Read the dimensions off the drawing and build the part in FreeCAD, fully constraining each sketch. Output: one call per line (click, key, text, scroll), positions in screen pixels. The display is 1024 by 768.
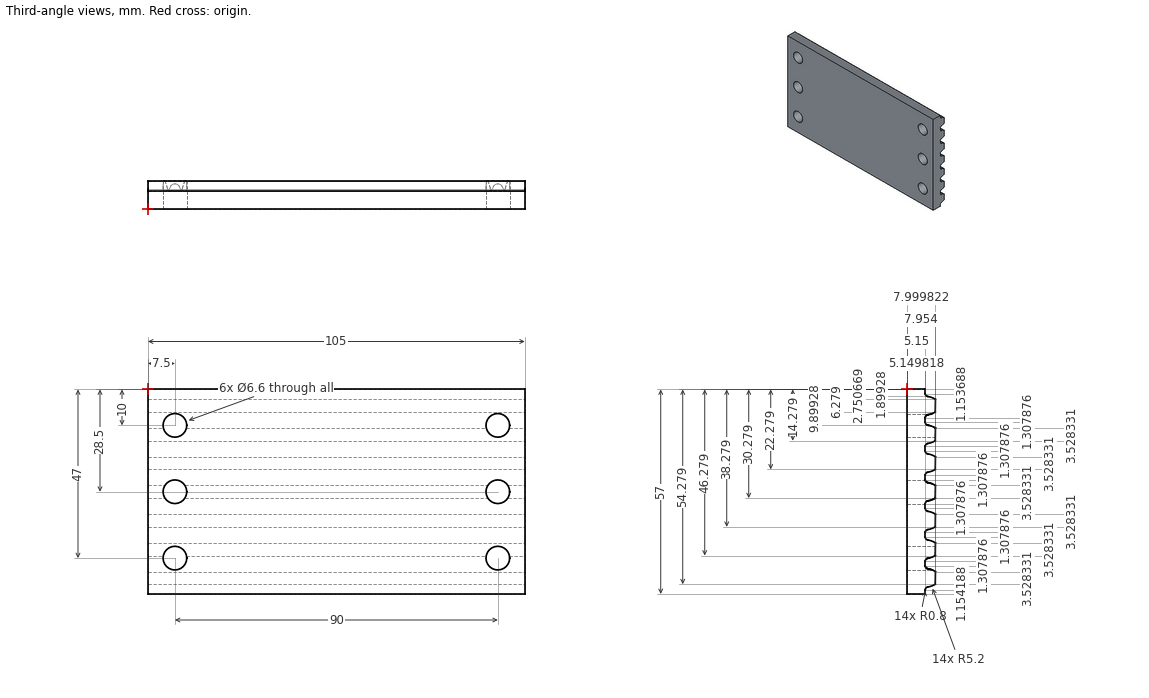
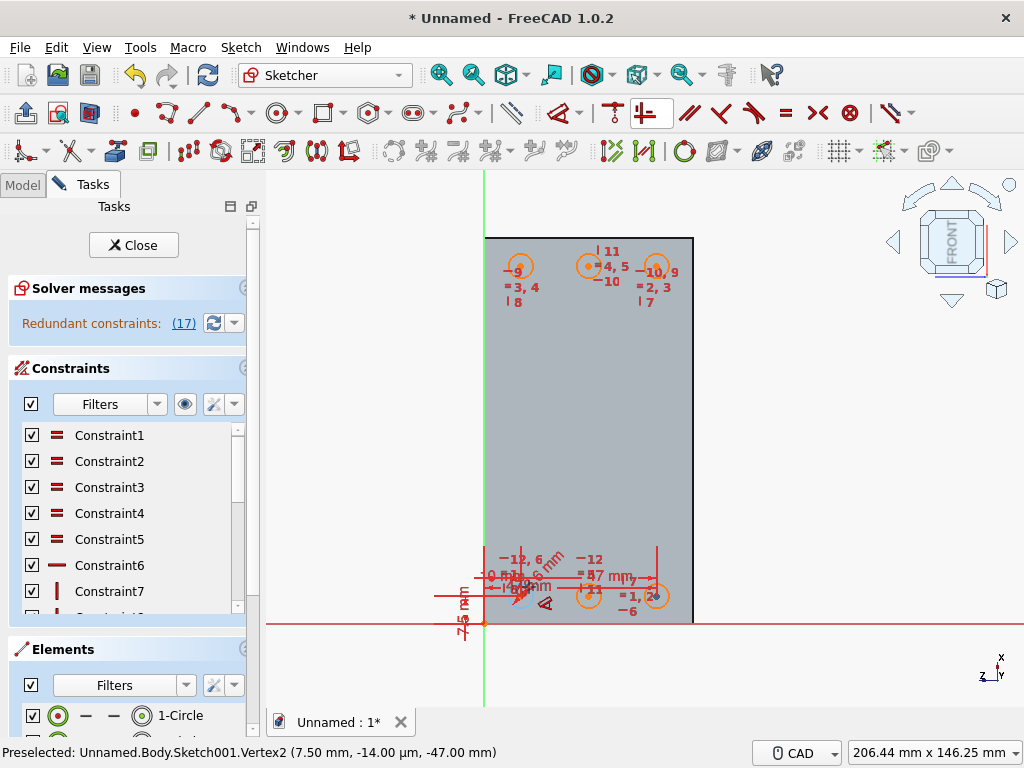
click(657, 266)
click(691, 431)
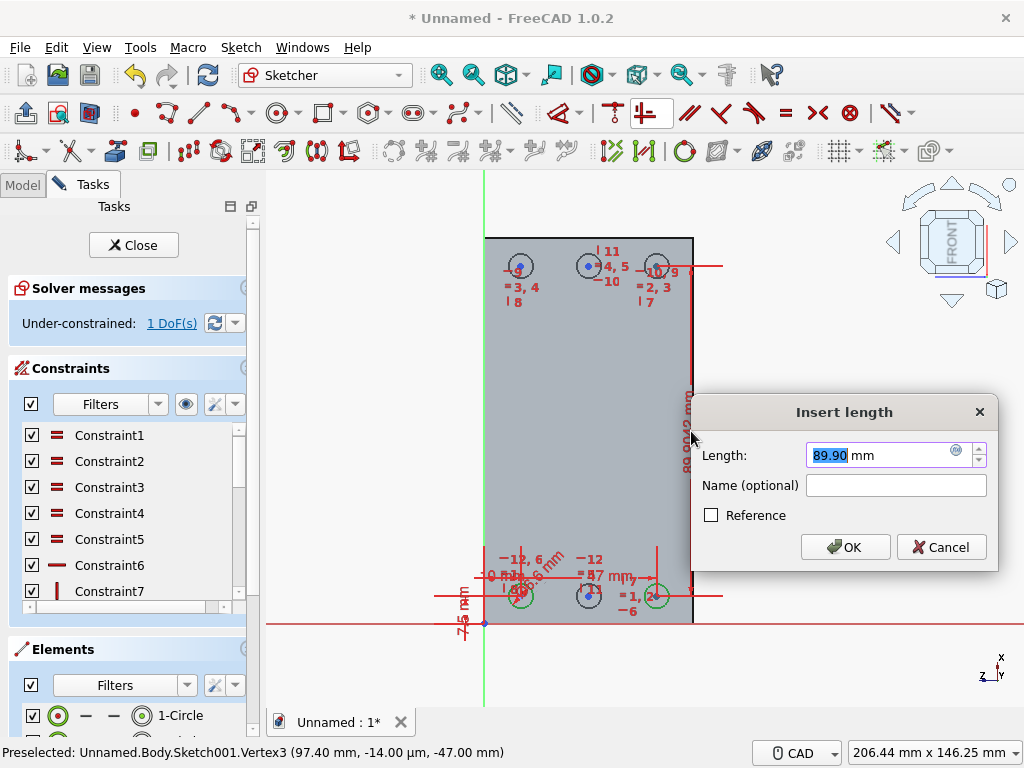
text(90)
key(Return)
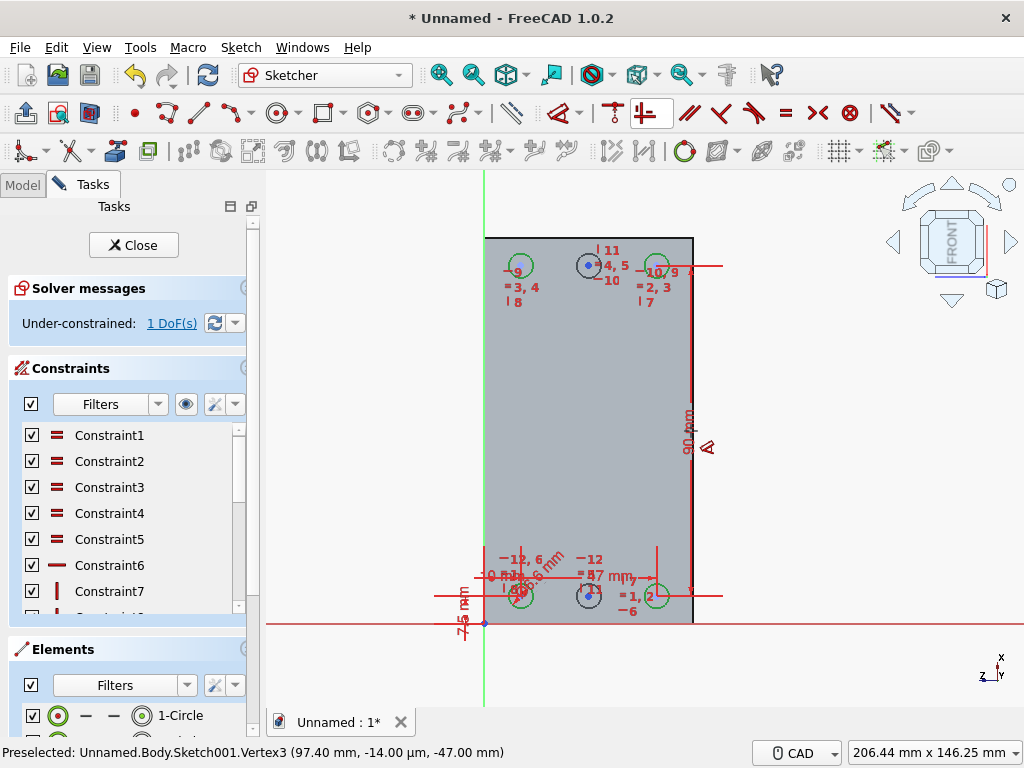
click(589, 266)
click(537, 658)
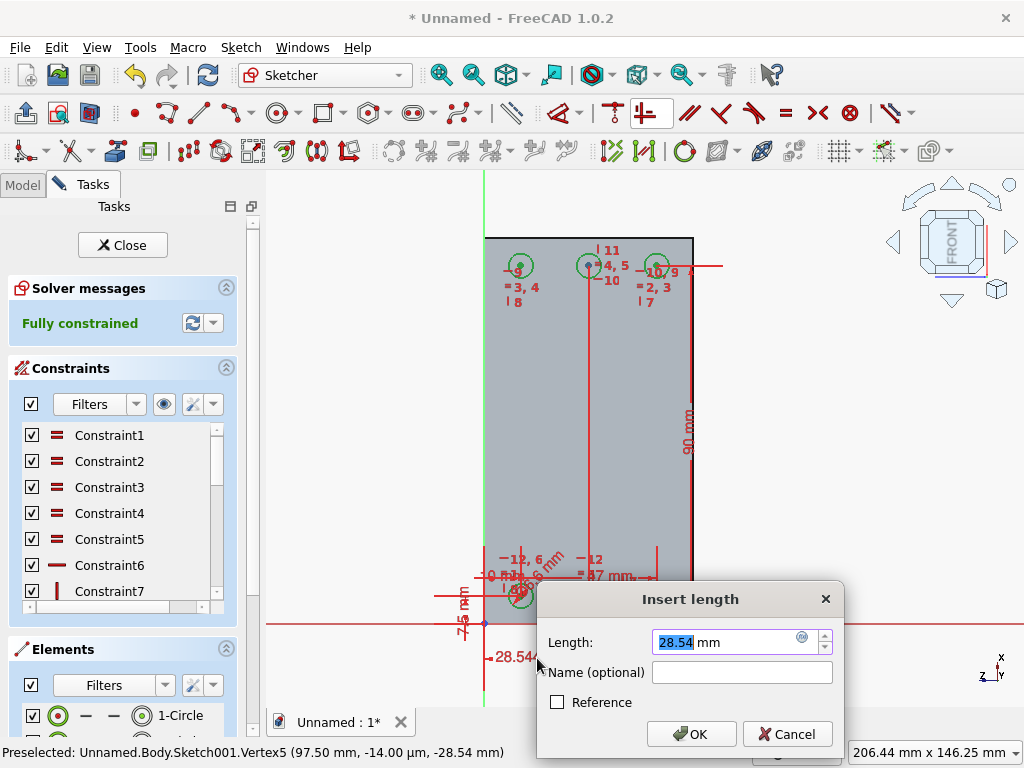
text(28.5)
key(Return)
key(Escape)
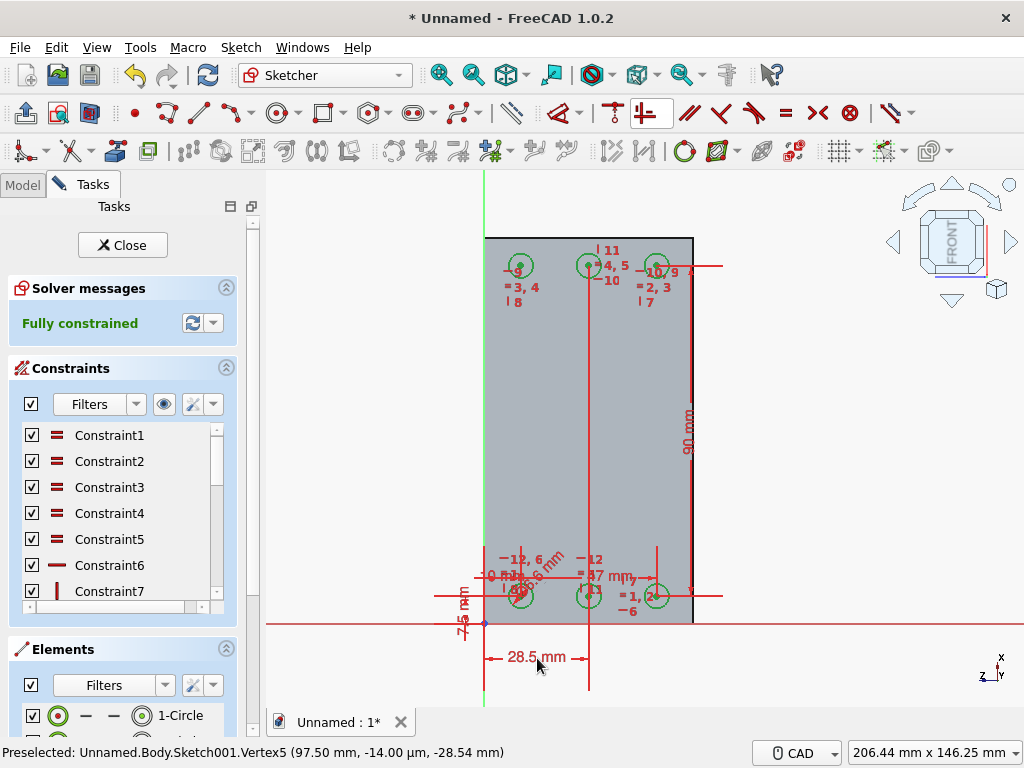
click(123, 245)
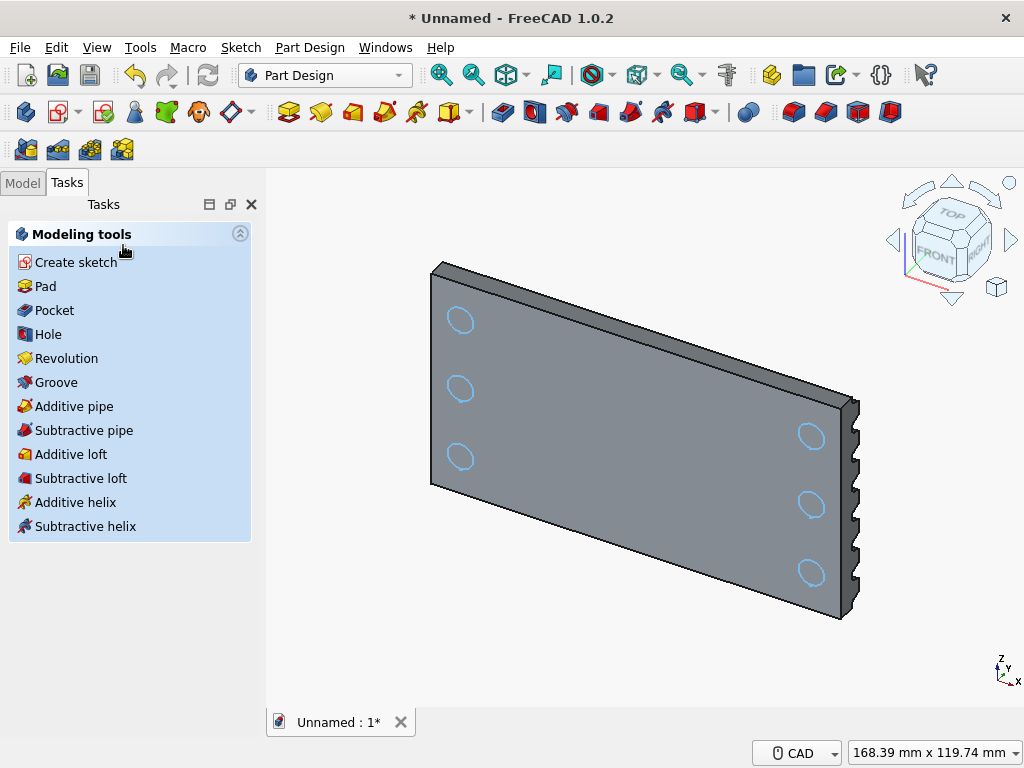
click(536, 112)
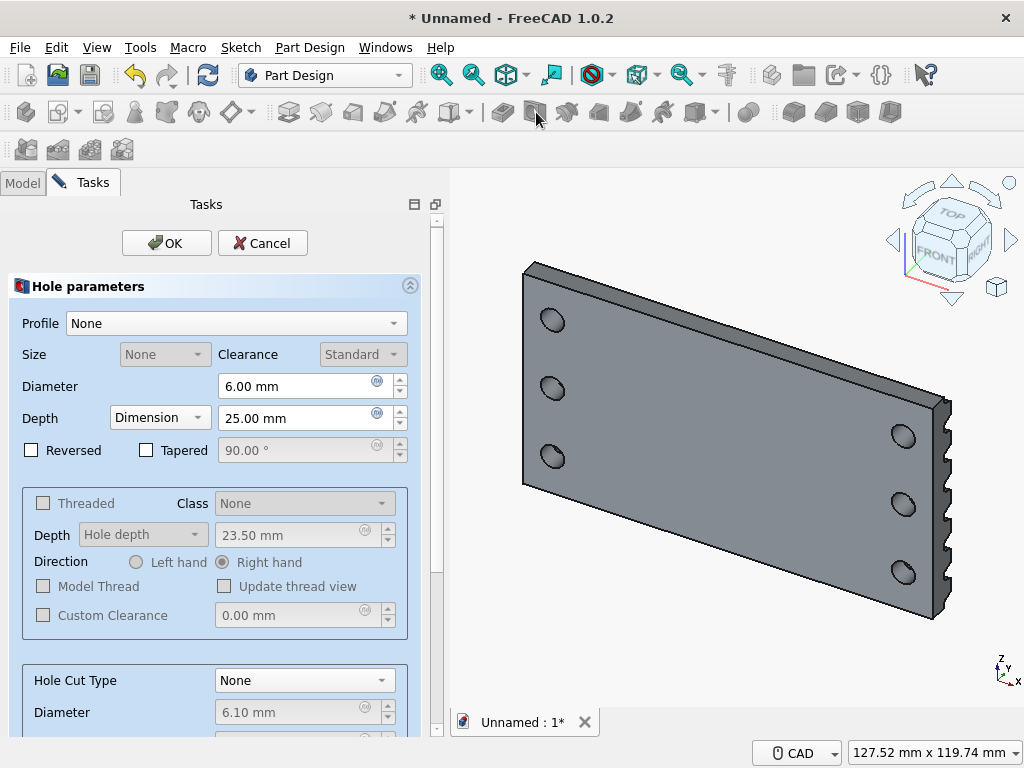
triple_click(305, 386)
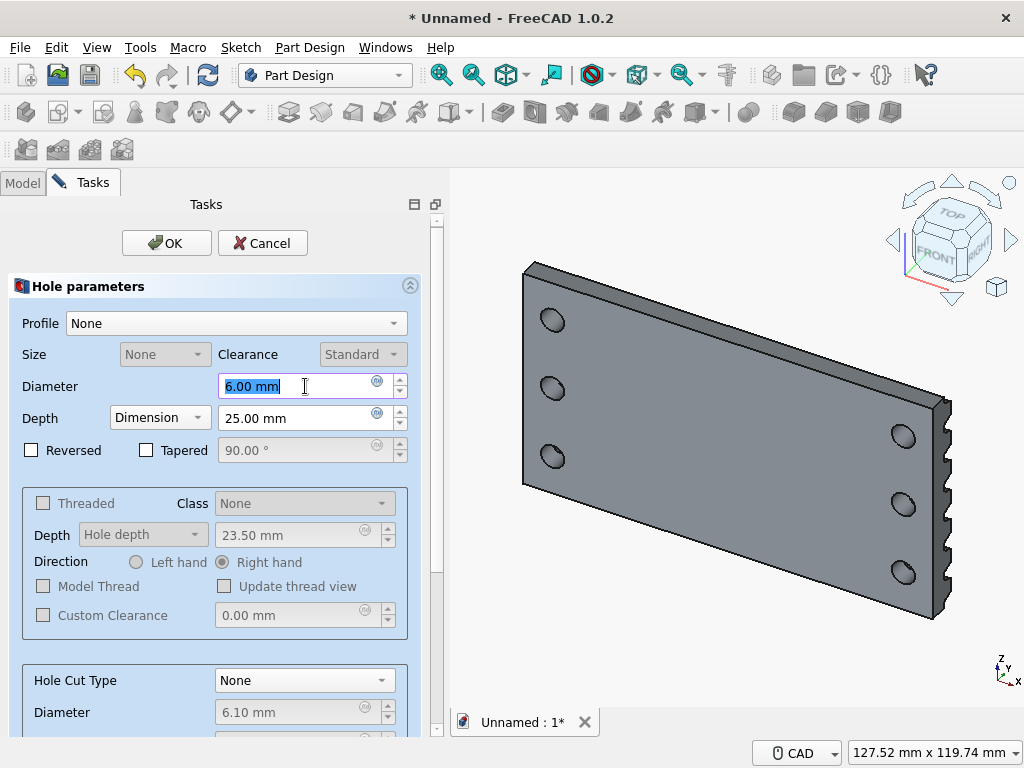
text(6.6)
key(Tab)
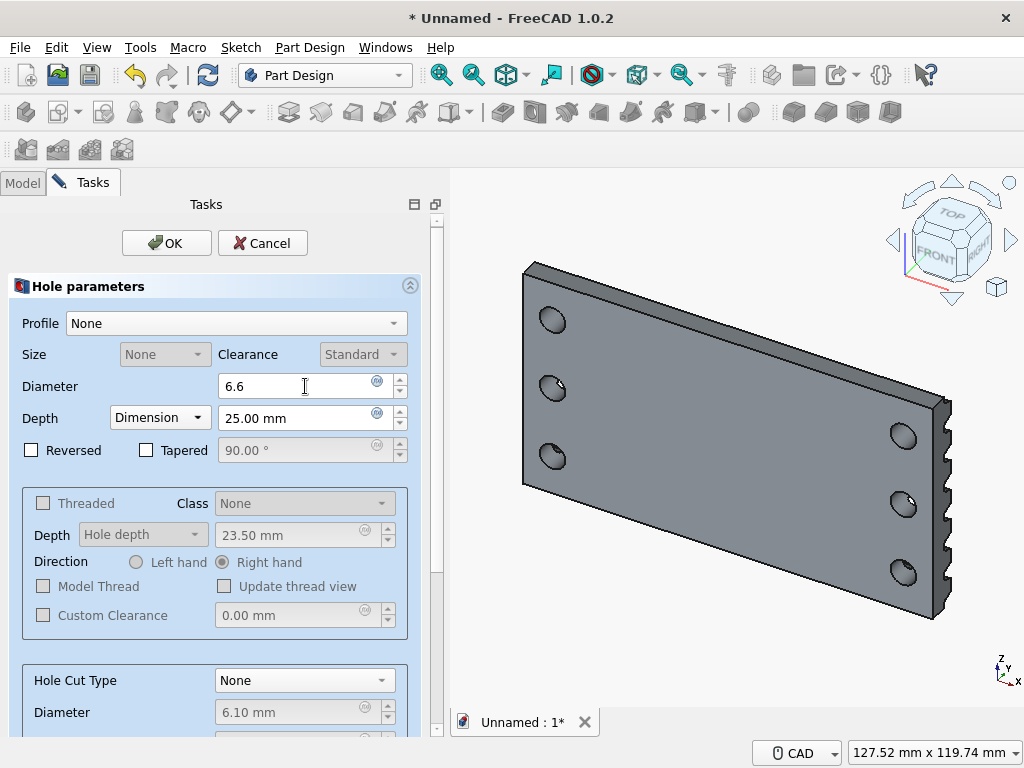
click(161, 418)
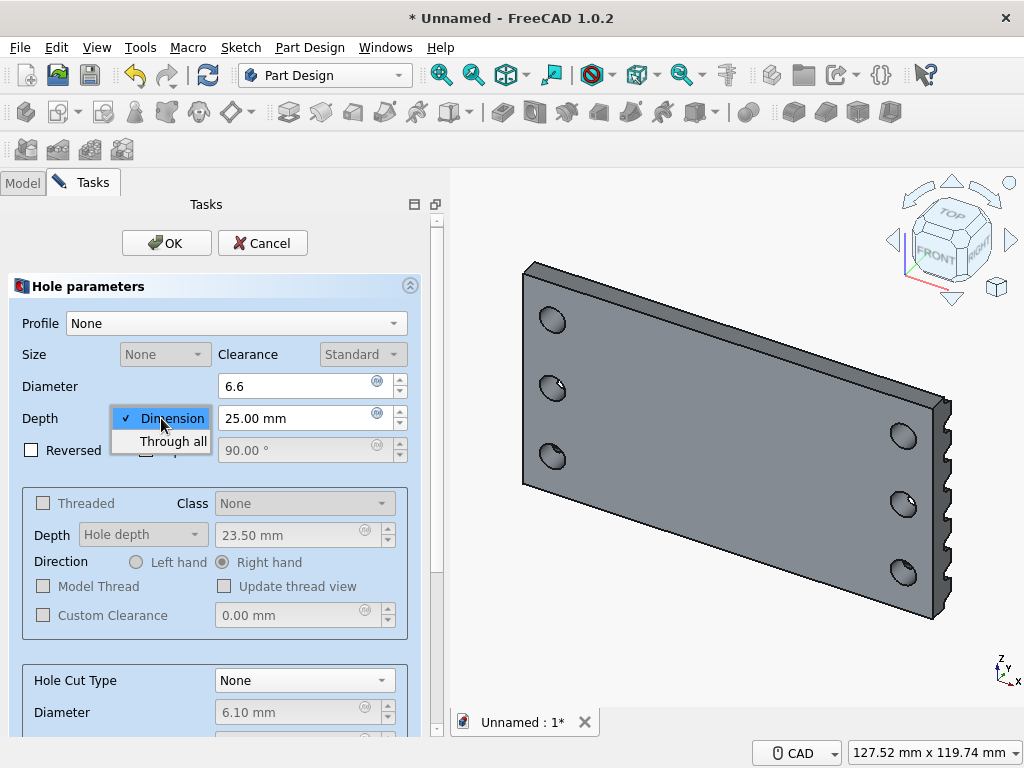
click(160, 442)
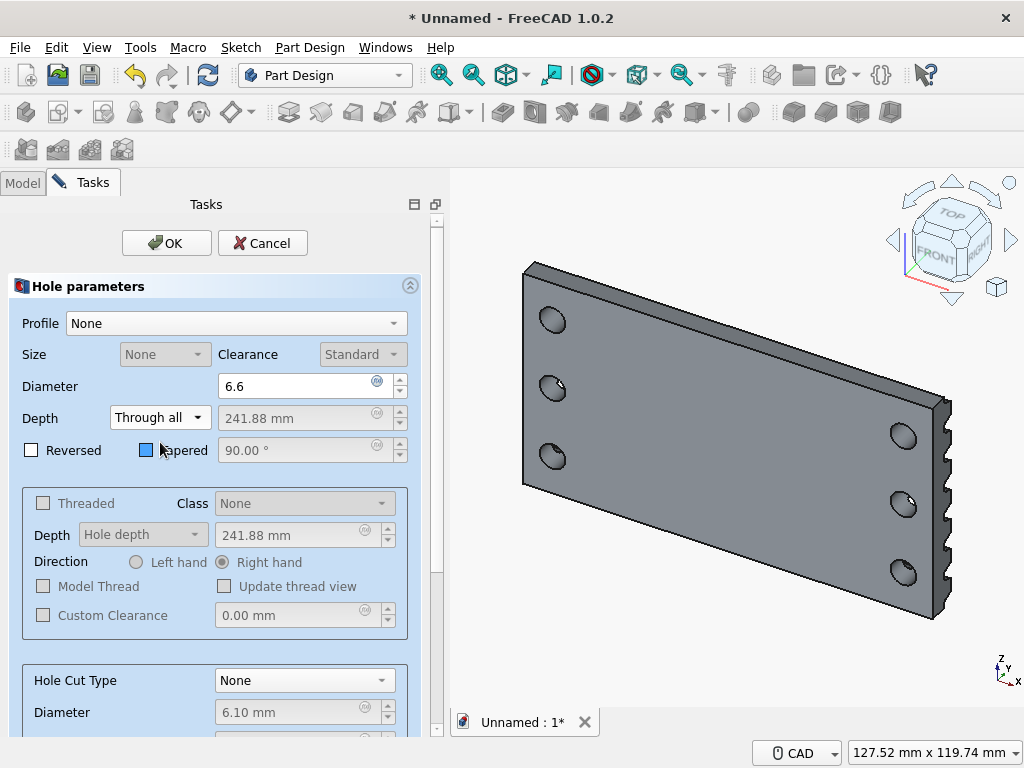
click(167, 243)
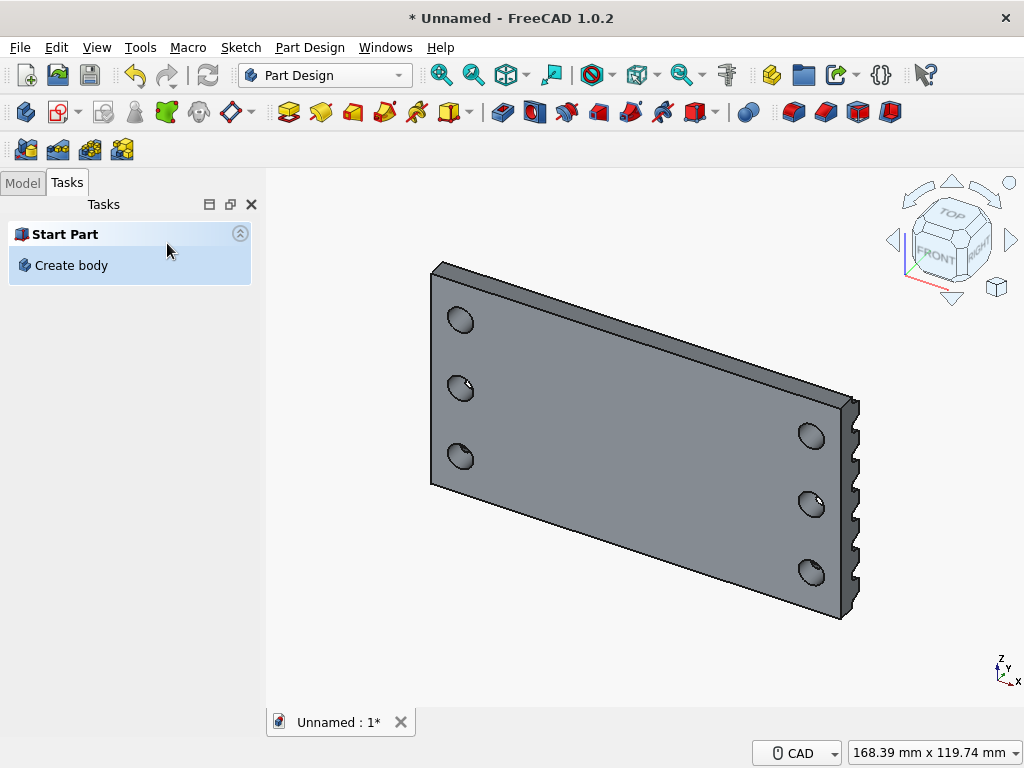
key(0)